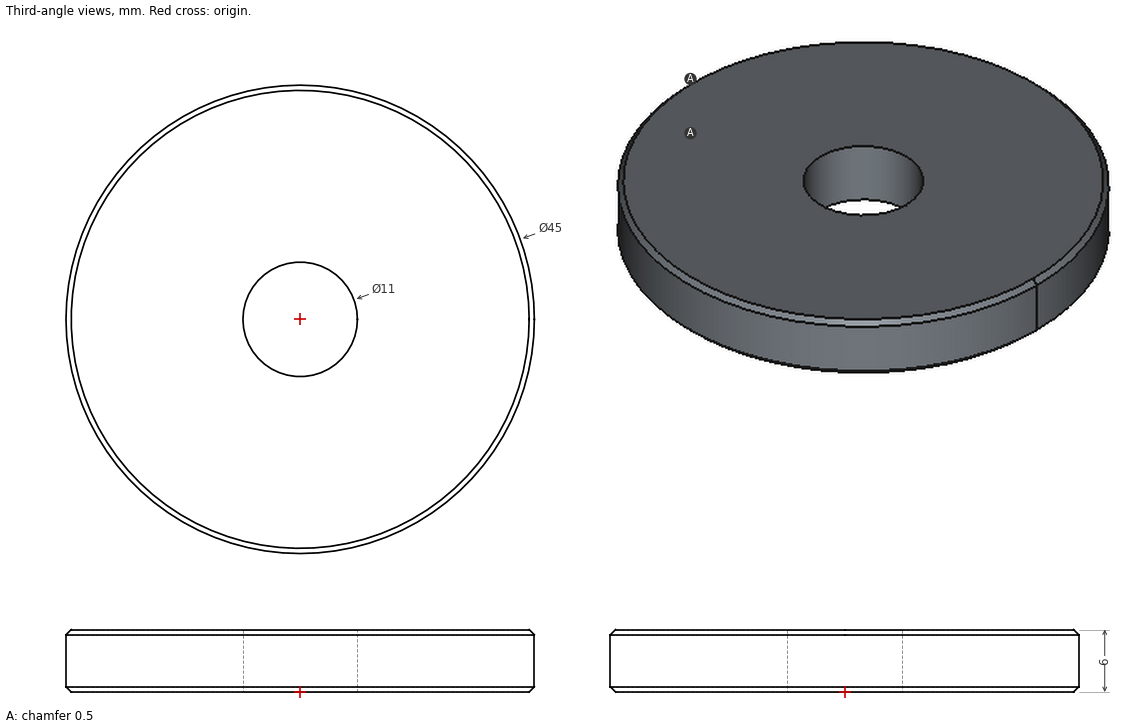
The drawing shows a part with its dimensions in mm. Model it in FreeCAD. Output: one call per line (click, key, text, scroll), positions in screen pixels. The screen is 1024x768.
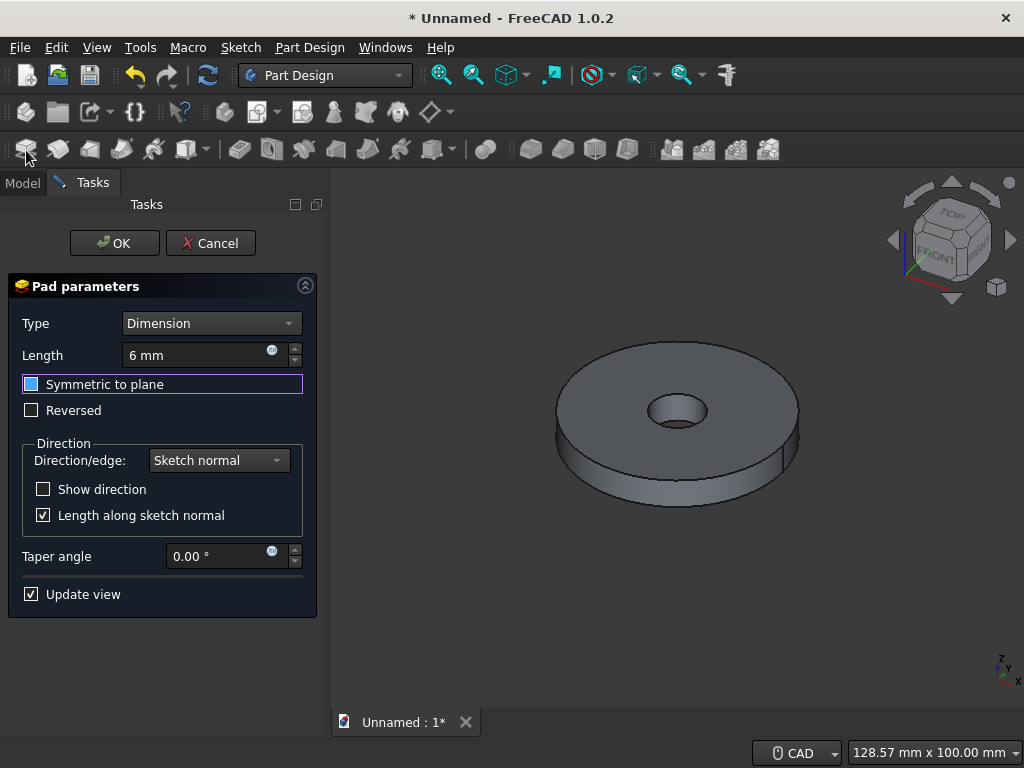
click(115, 243)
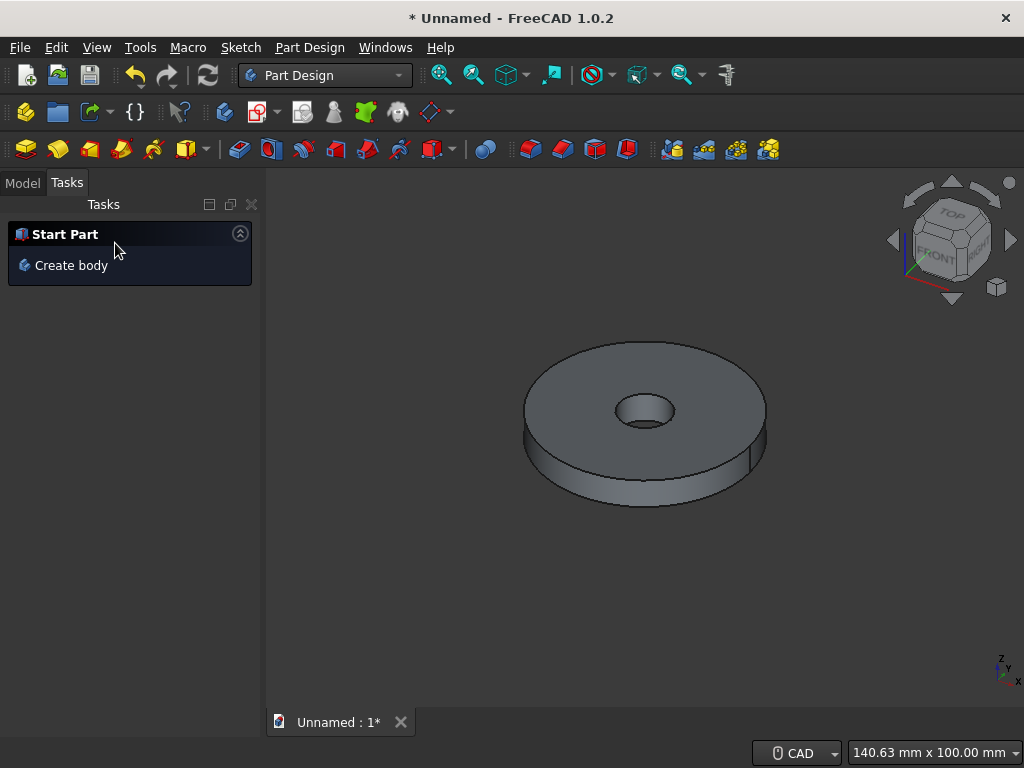
click(442, 76)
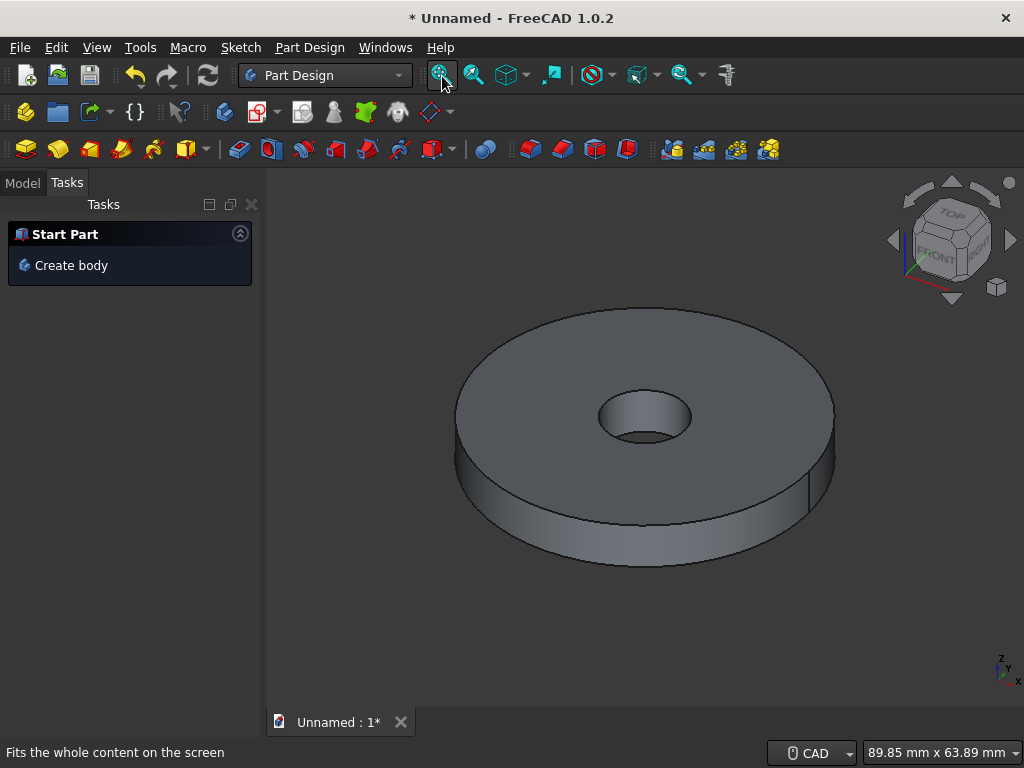
click(456, 427)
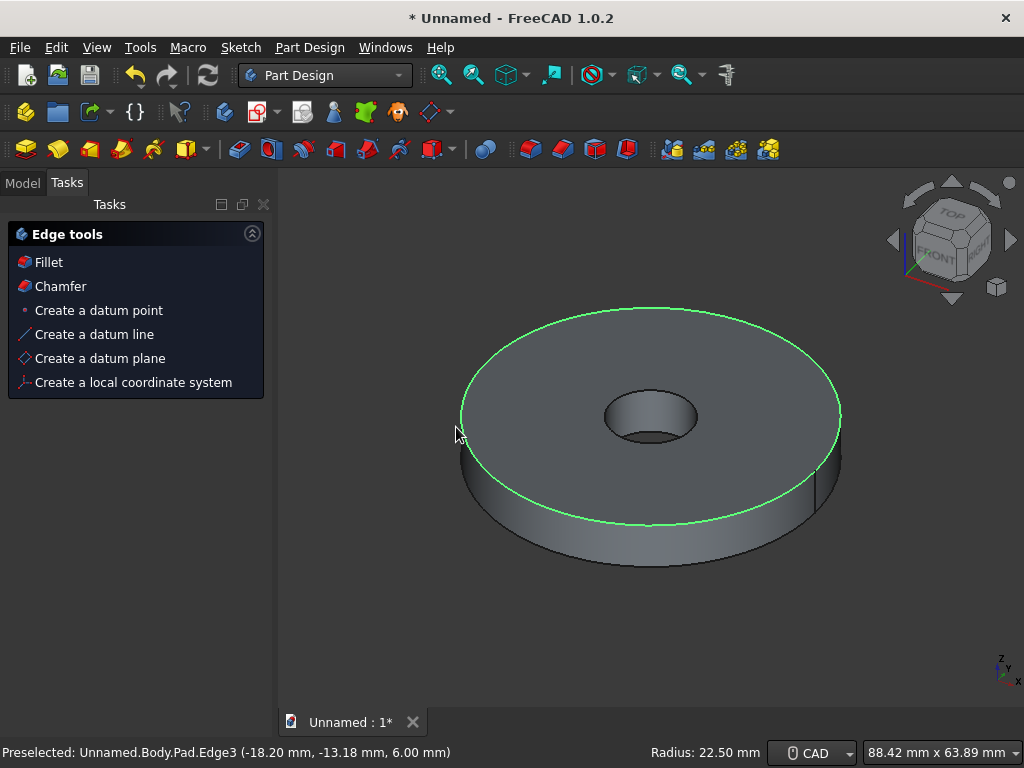
key(0)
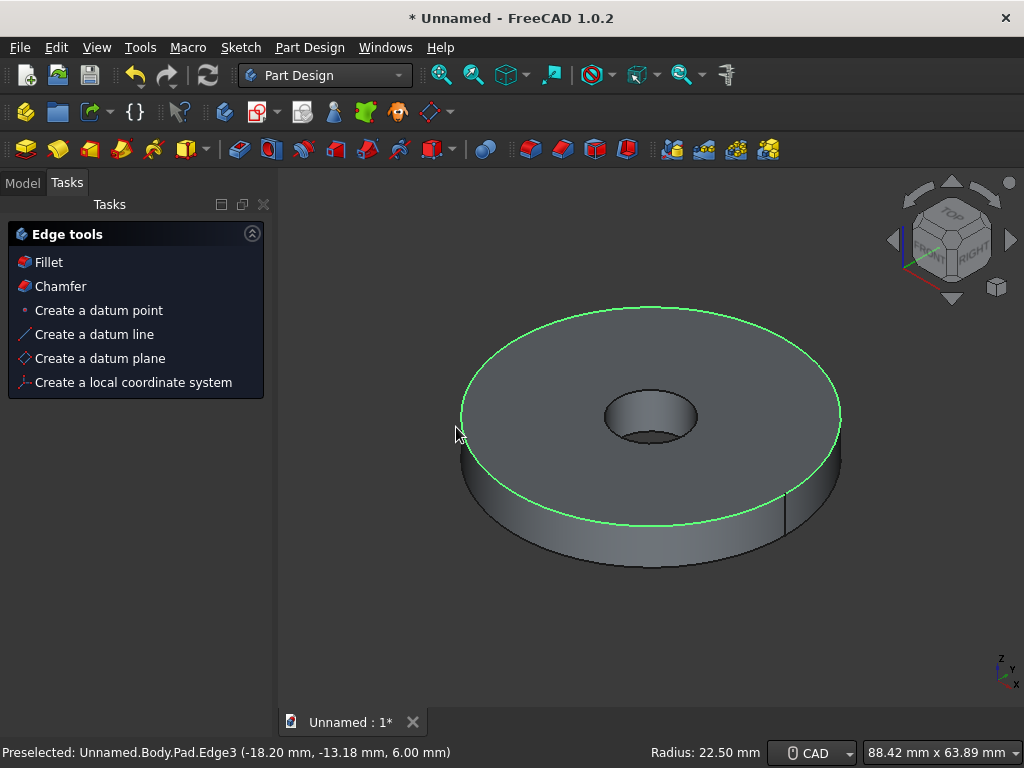
key(2)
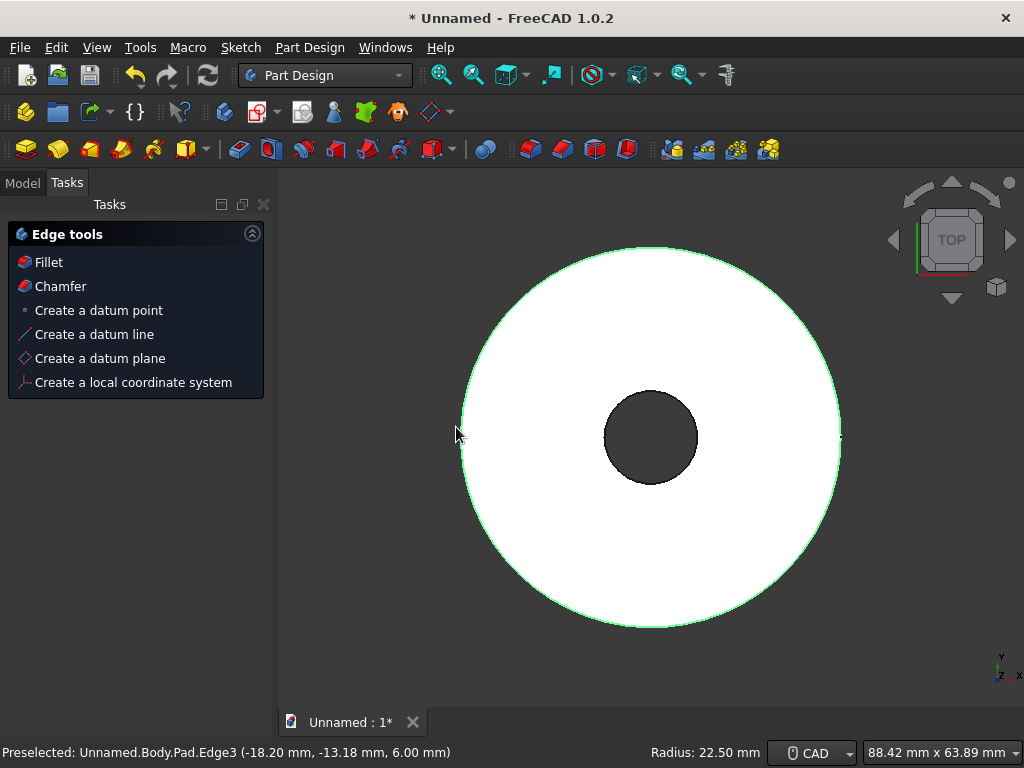
key(1)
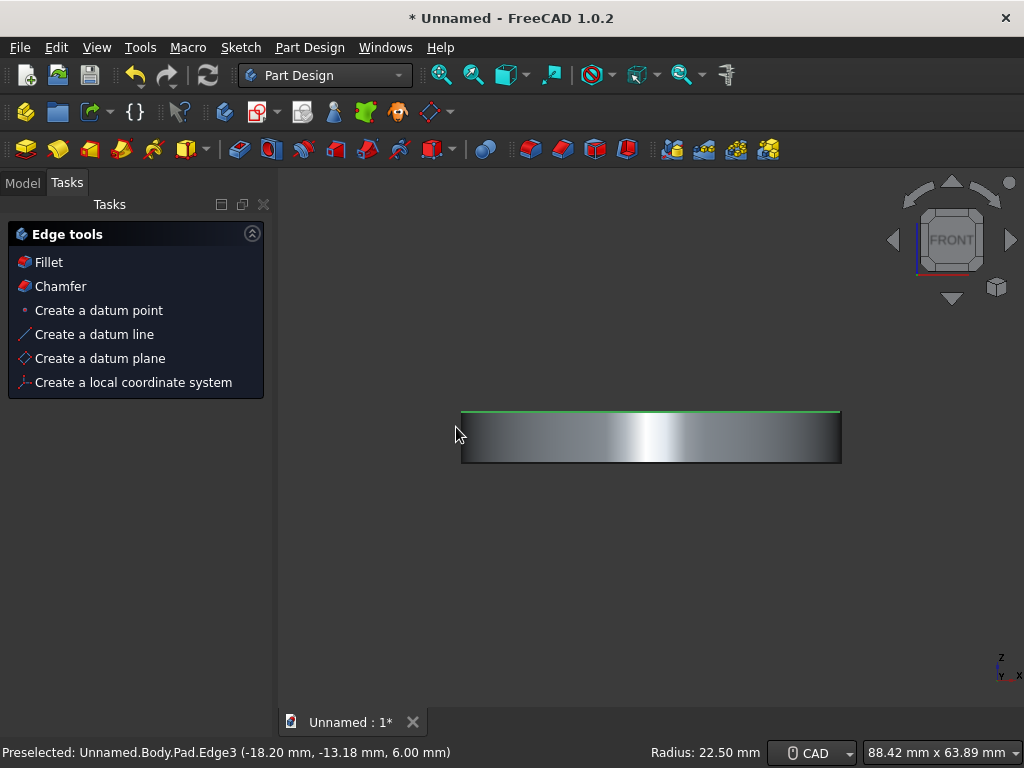
click(497, 462, ctrl)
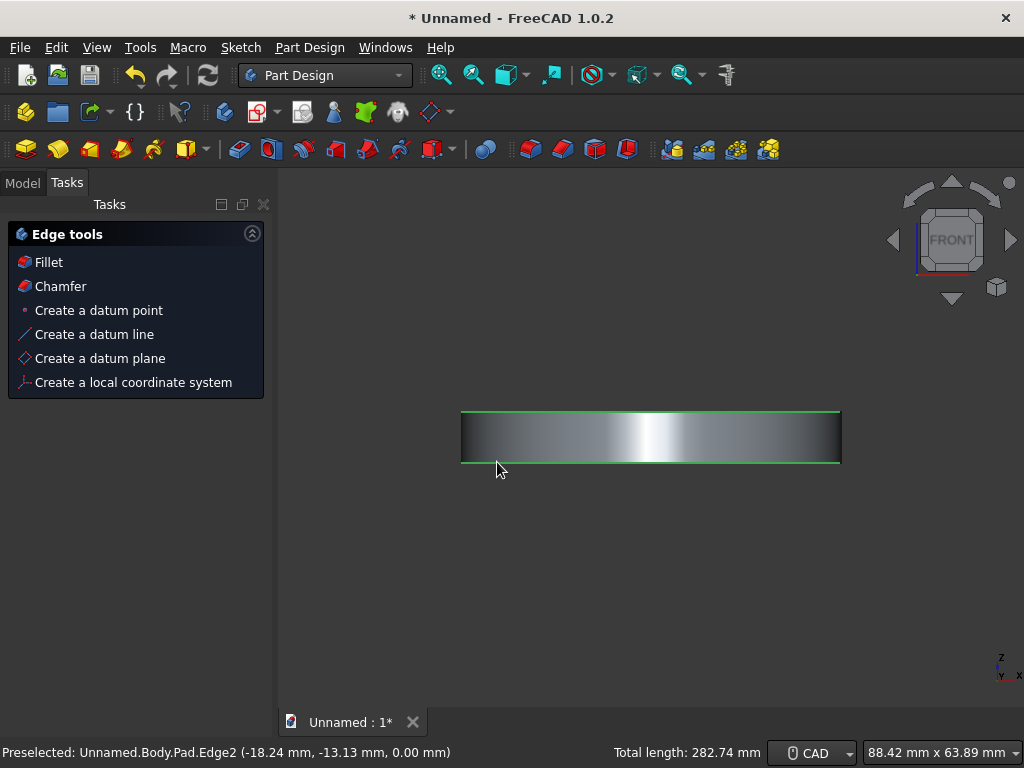
click(564, 150)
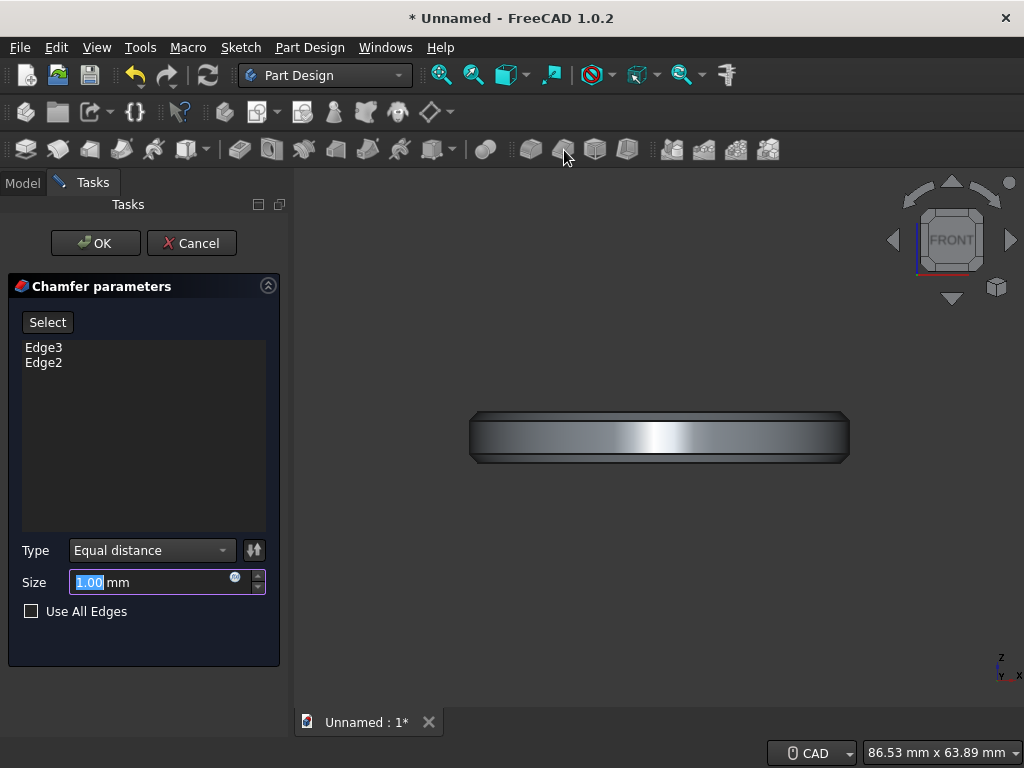
text(0.5)
key(Tab)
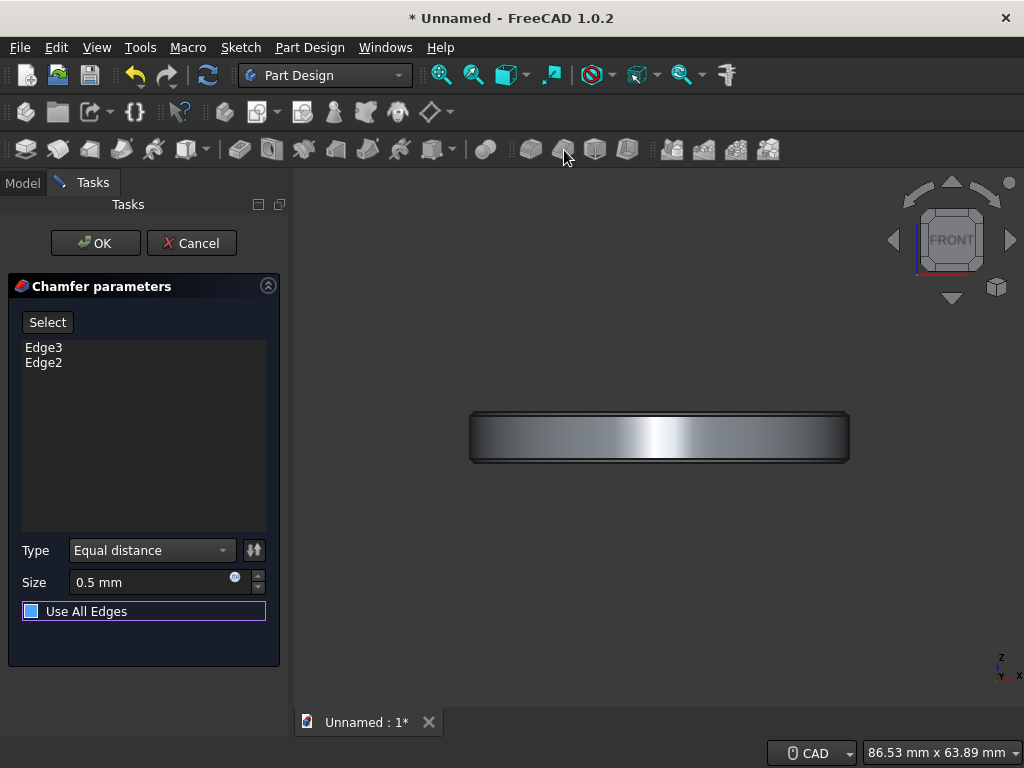
click(96, 243)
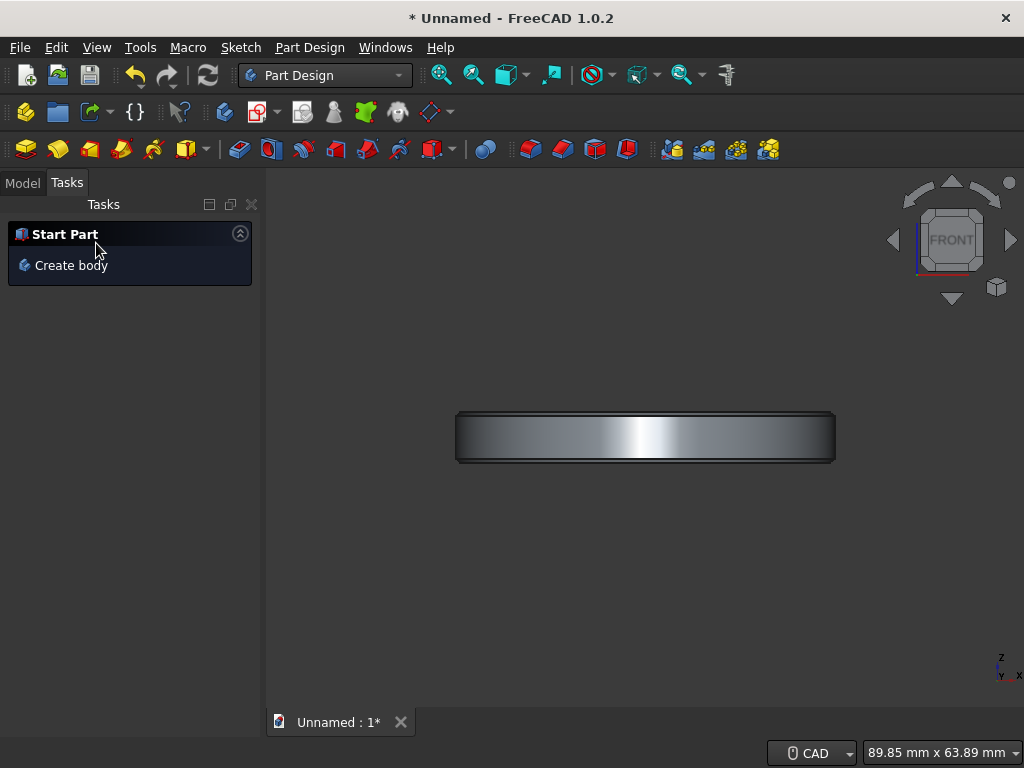
key(0)